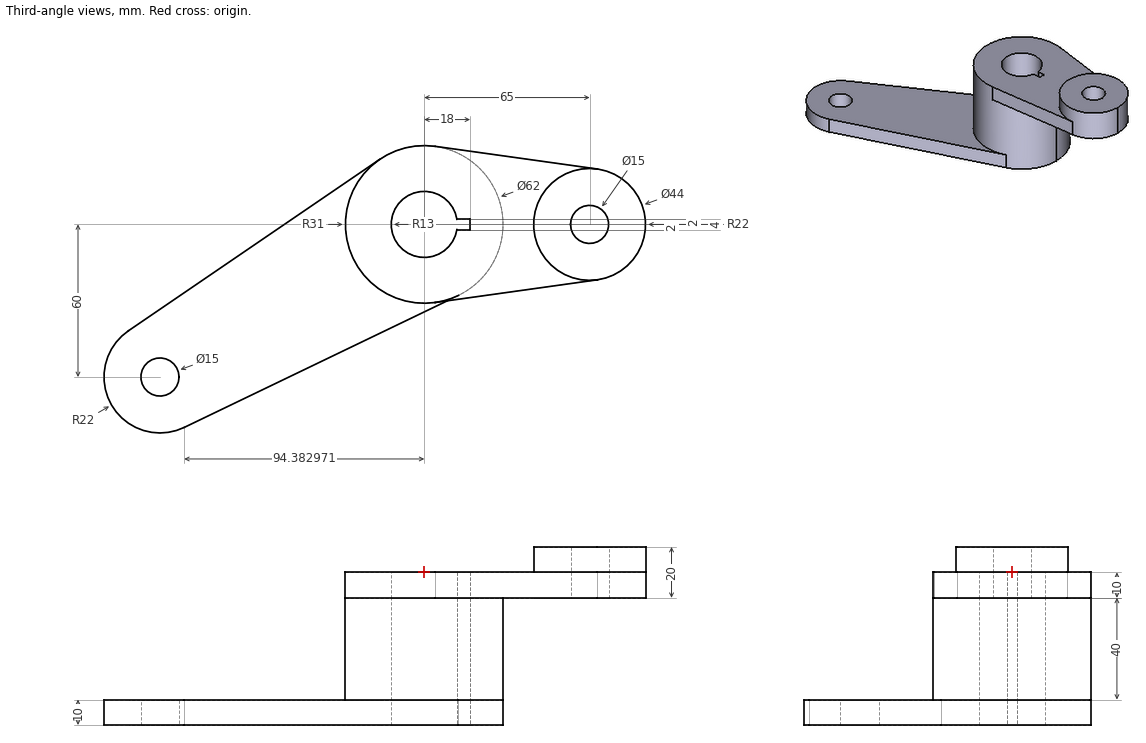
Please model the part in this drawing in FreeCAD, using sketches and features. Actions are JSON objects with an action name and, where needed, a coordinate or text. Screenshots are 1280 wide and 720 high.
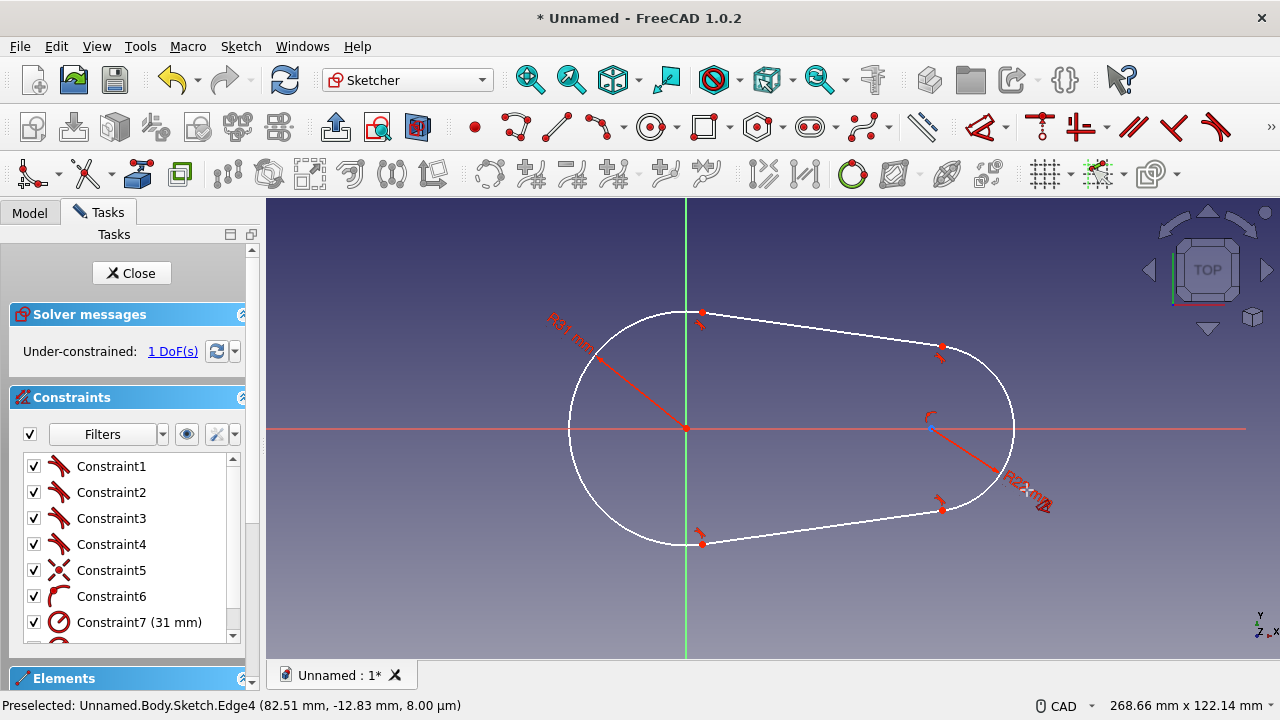
{"action": "left_click", "coordinate": [931, 428]}
{"action": "left_click", "coordinate": [809, 462]}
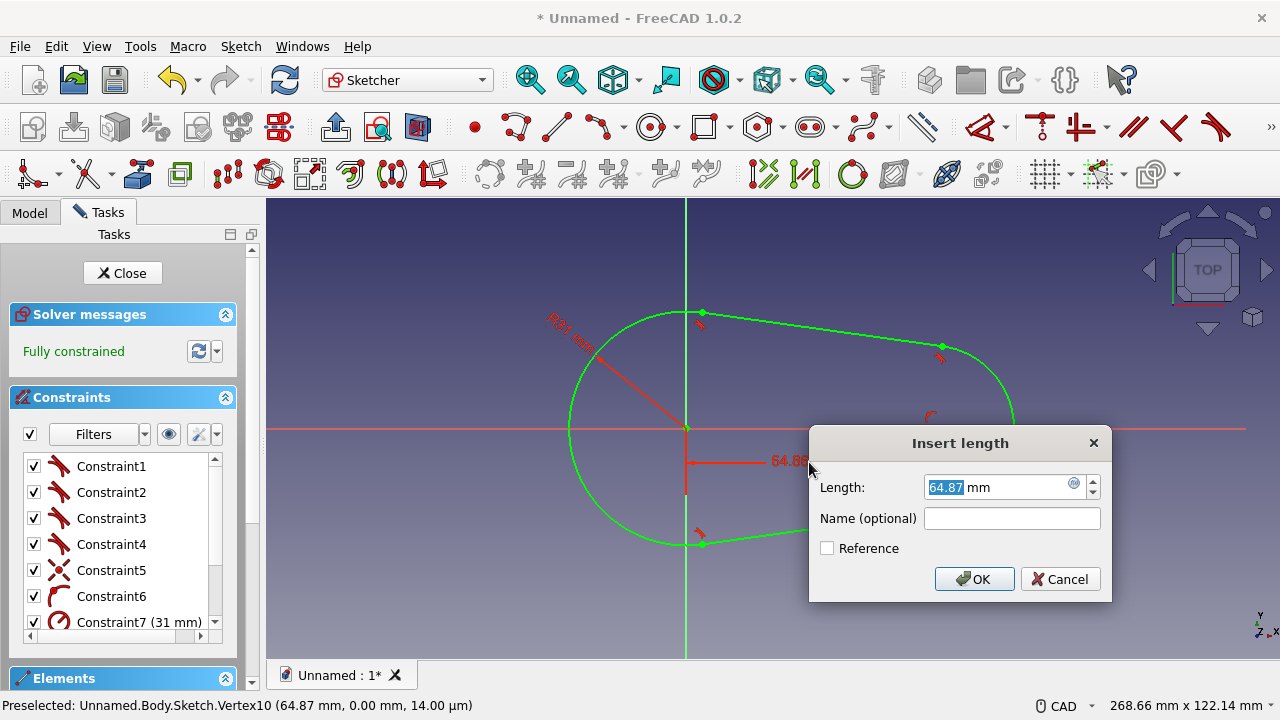
{"action": "type", "text": "65"}
{"action": "key", "text": "Return"}
{"action": "key", "text": "Escape"}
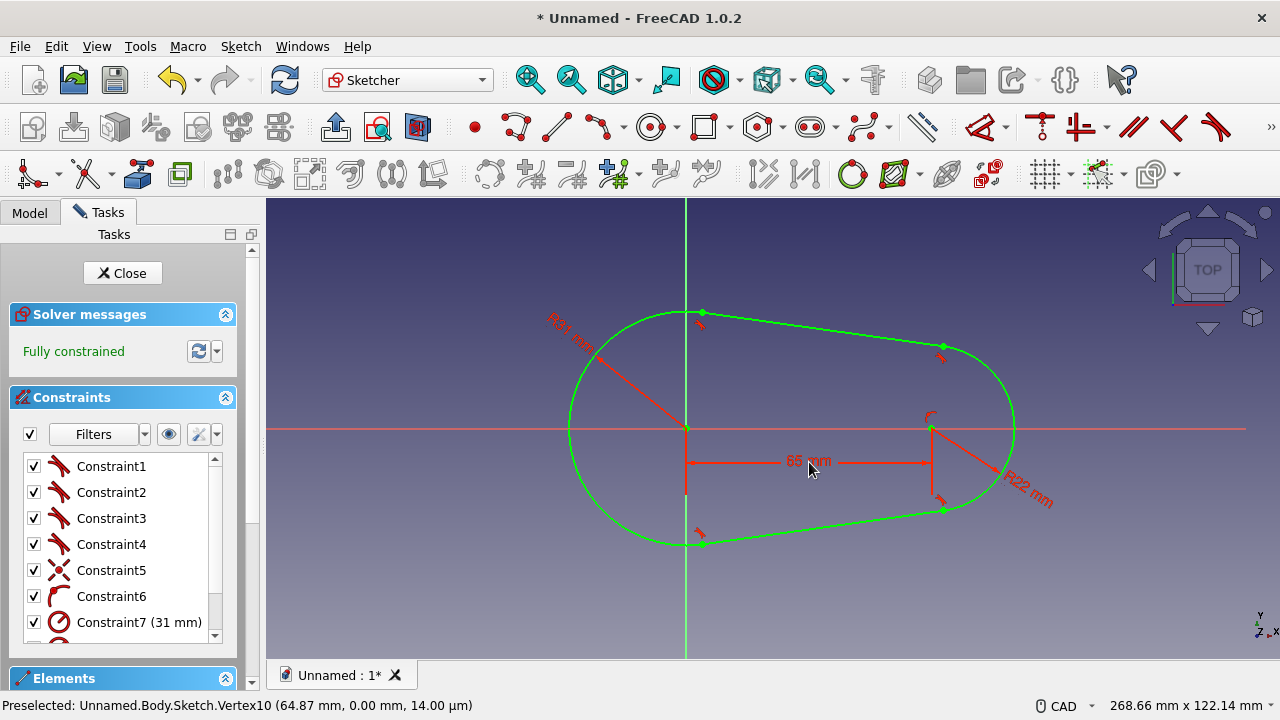
{"action": "left_click", "coordinate": [123, 273]}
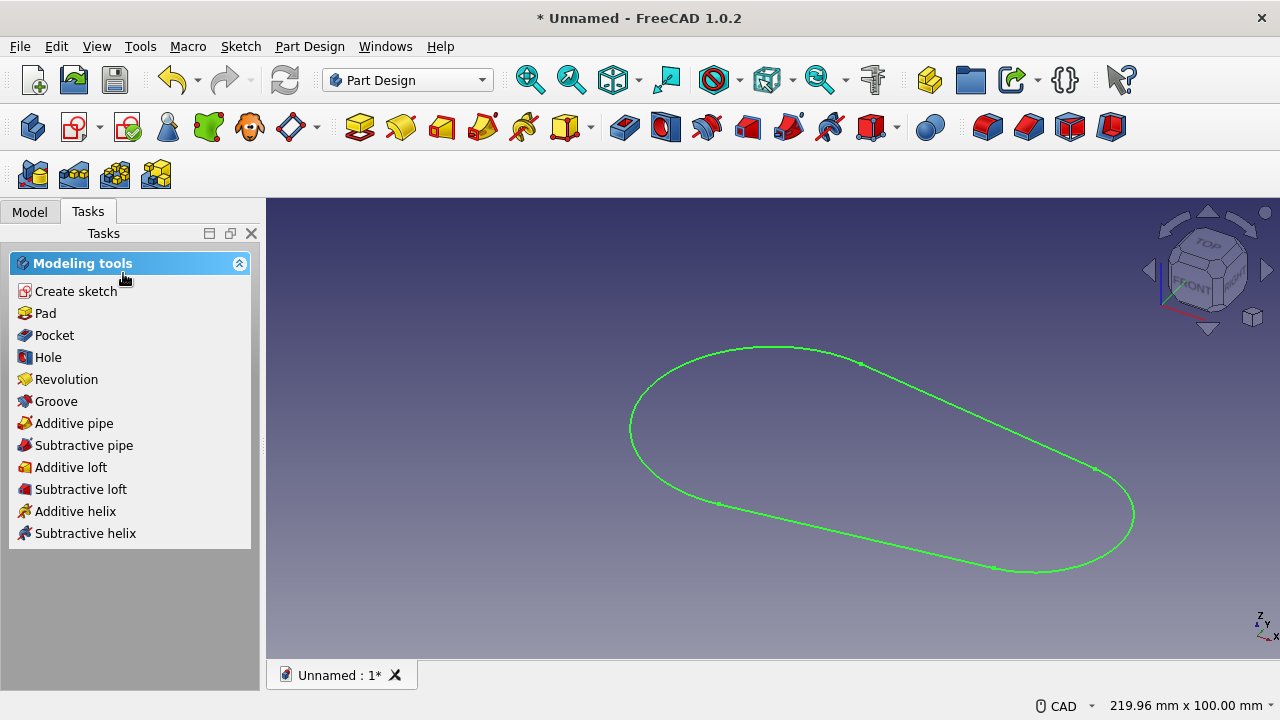
{"action": "left_click", "coordinate": [360, 128]}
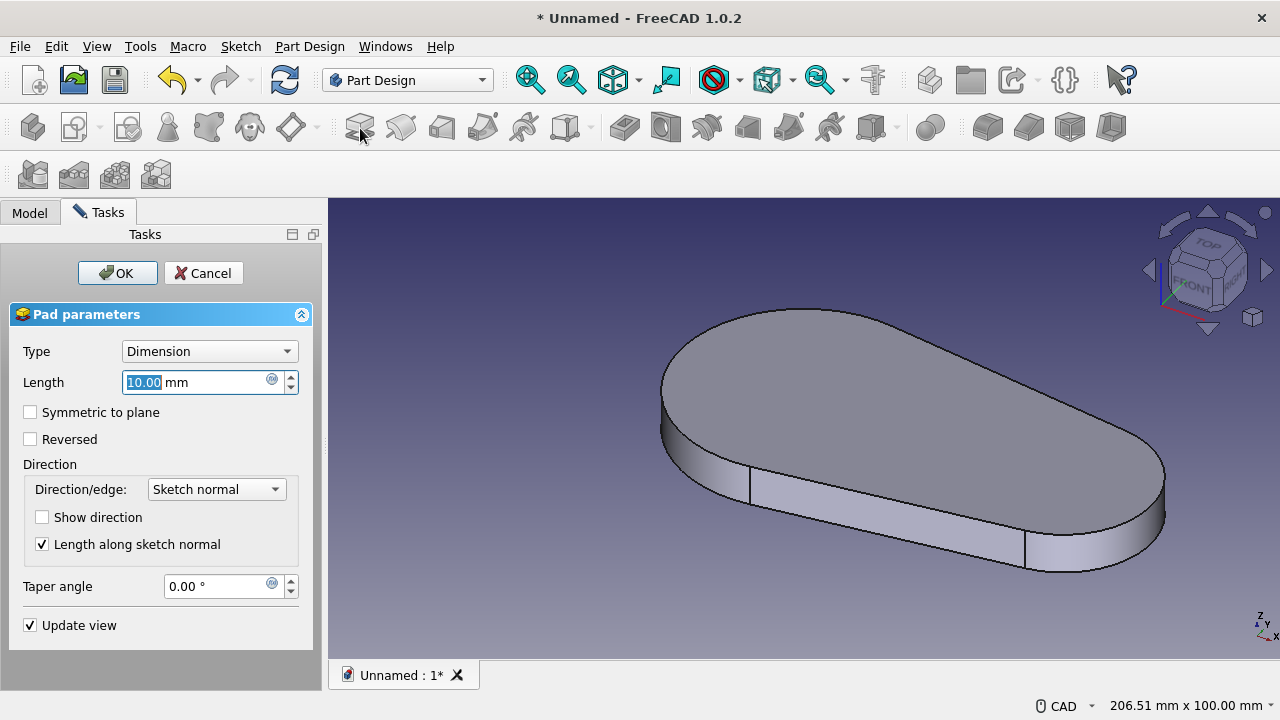
{"action": "type", "text": "10"}
{"action": "key", "text": "Tab"}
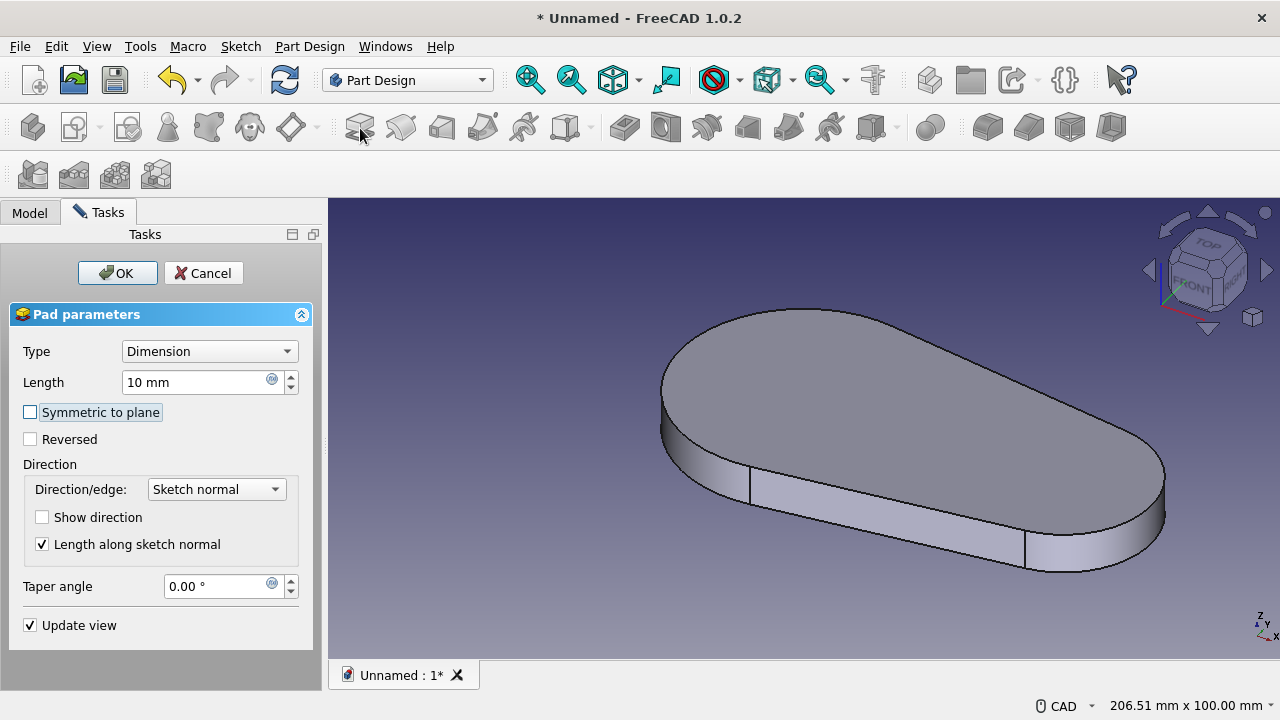
{"action": "left_click", "coordinate": [31, 439]}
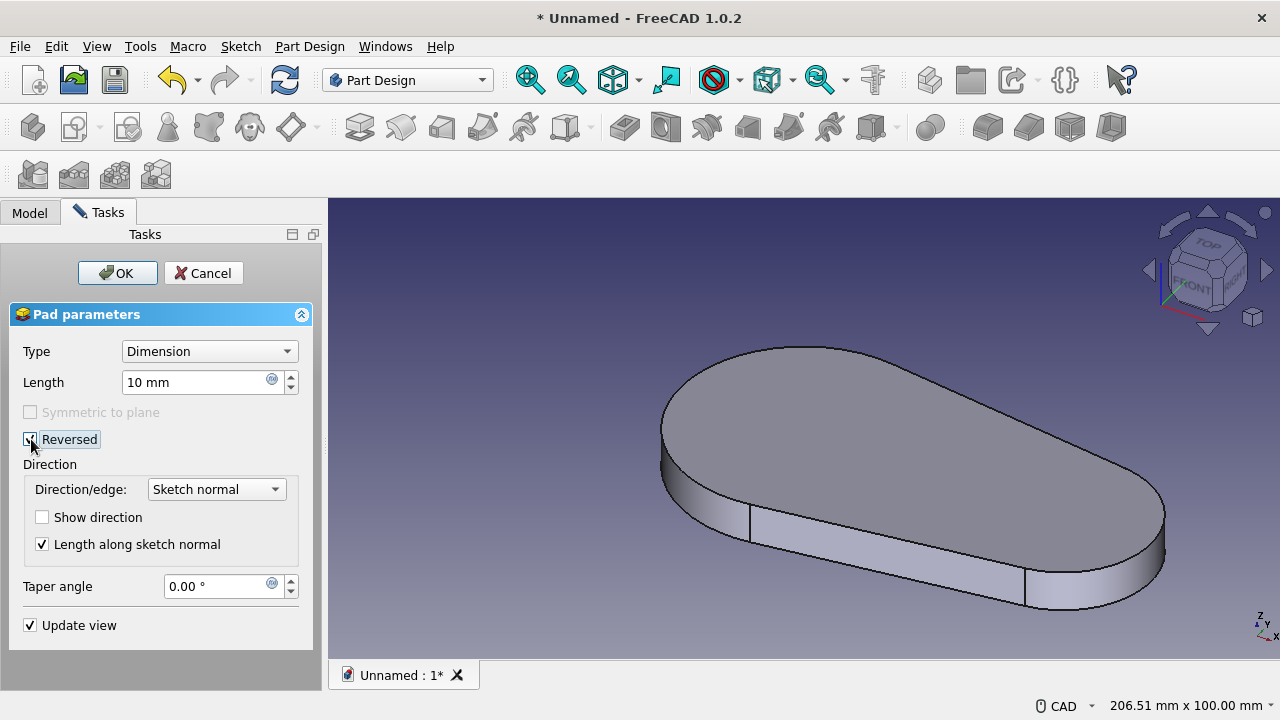
{"action": "left_click", "coordinate": [118, 273]}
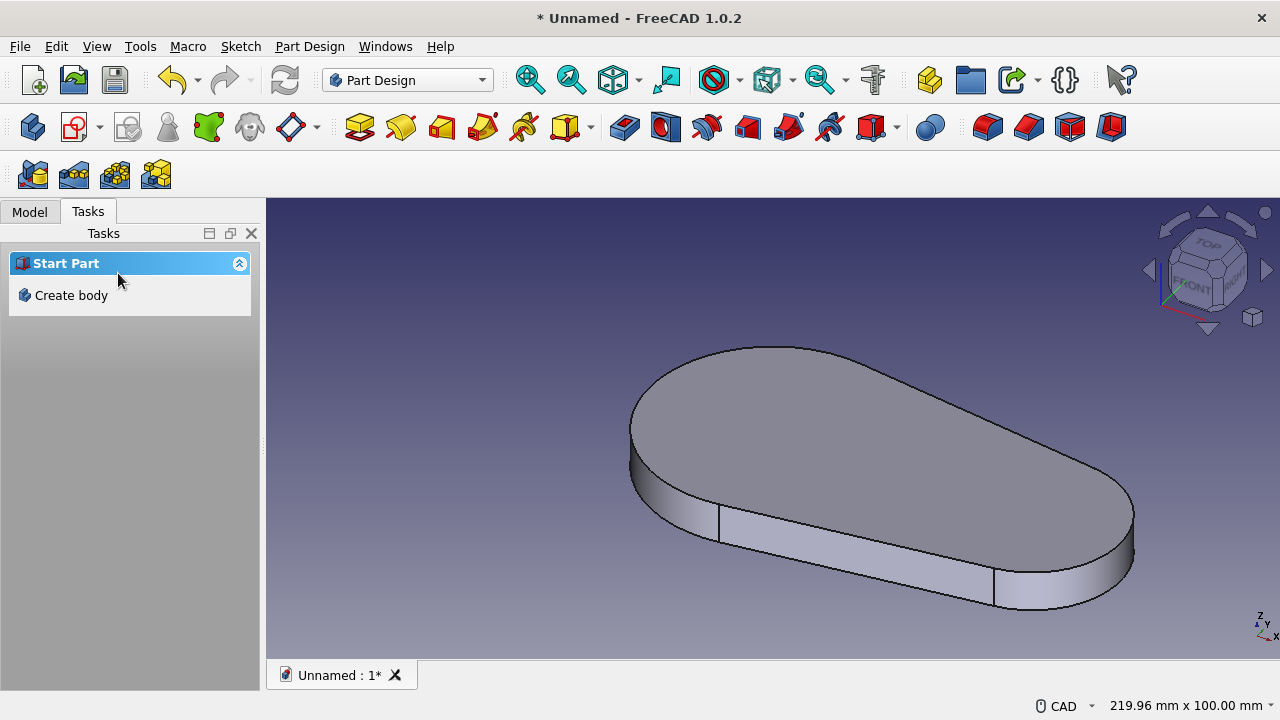
{"action": "left_click", "coordinate": [30, 212]}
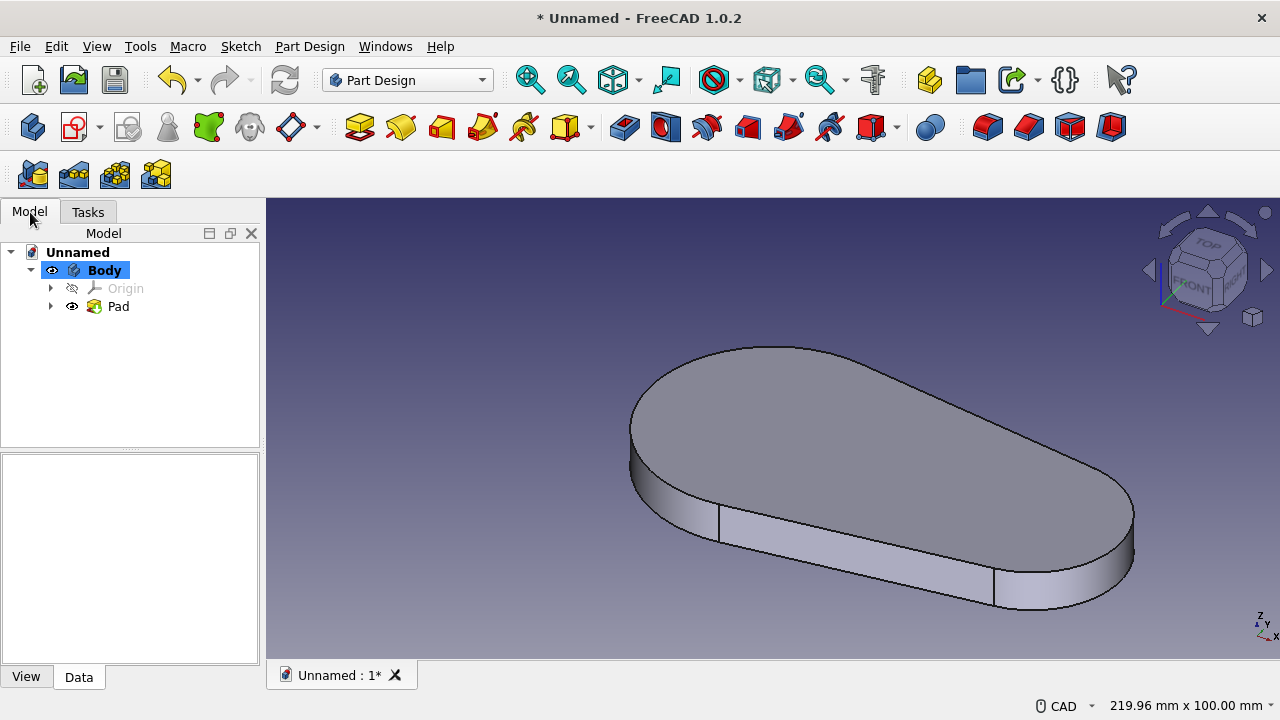
{"action": "left_click", "coordinate": [51, 288]}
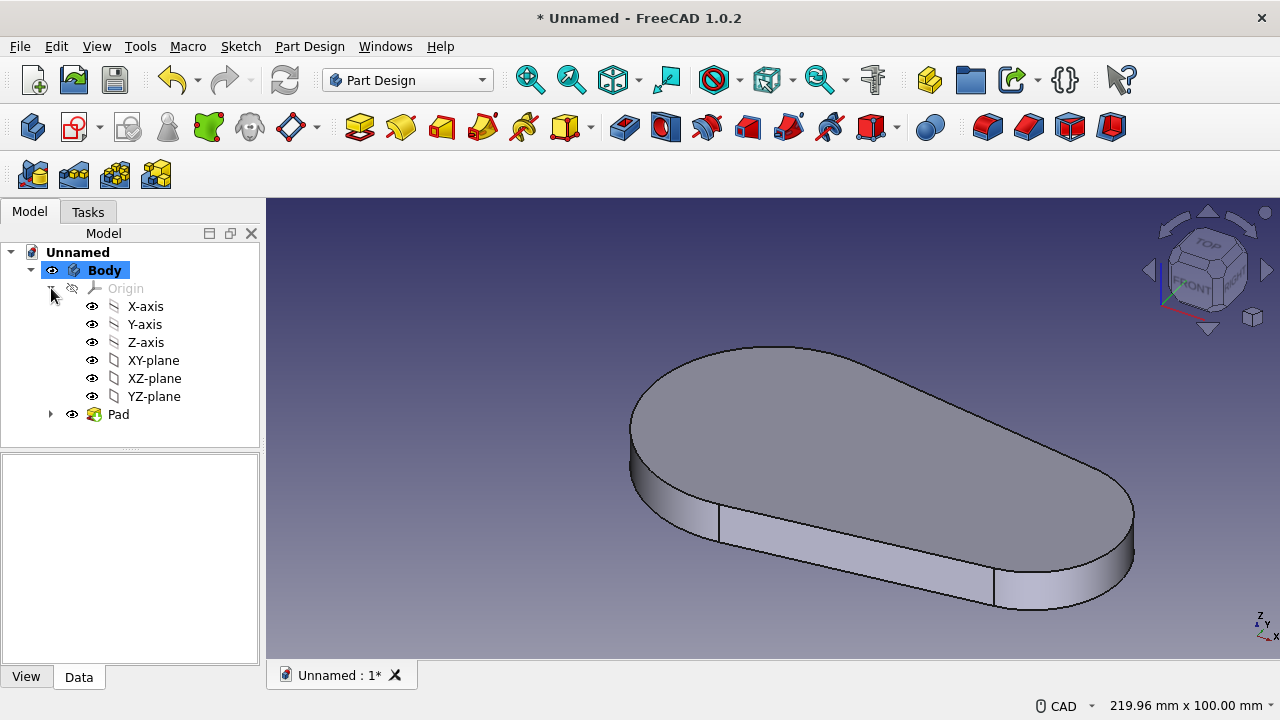
{"action": "left_click", "coordinate": [137, 360]}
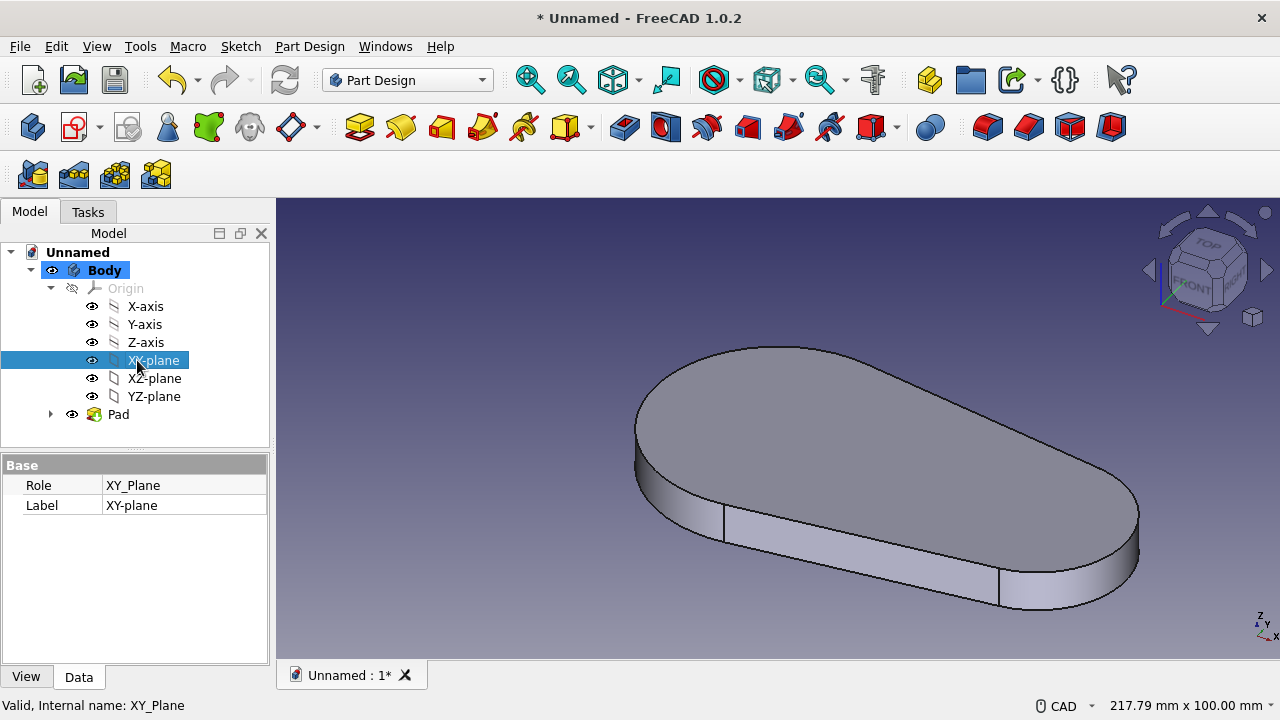
{"action": "left_click", "coordinate": [290, 128]}